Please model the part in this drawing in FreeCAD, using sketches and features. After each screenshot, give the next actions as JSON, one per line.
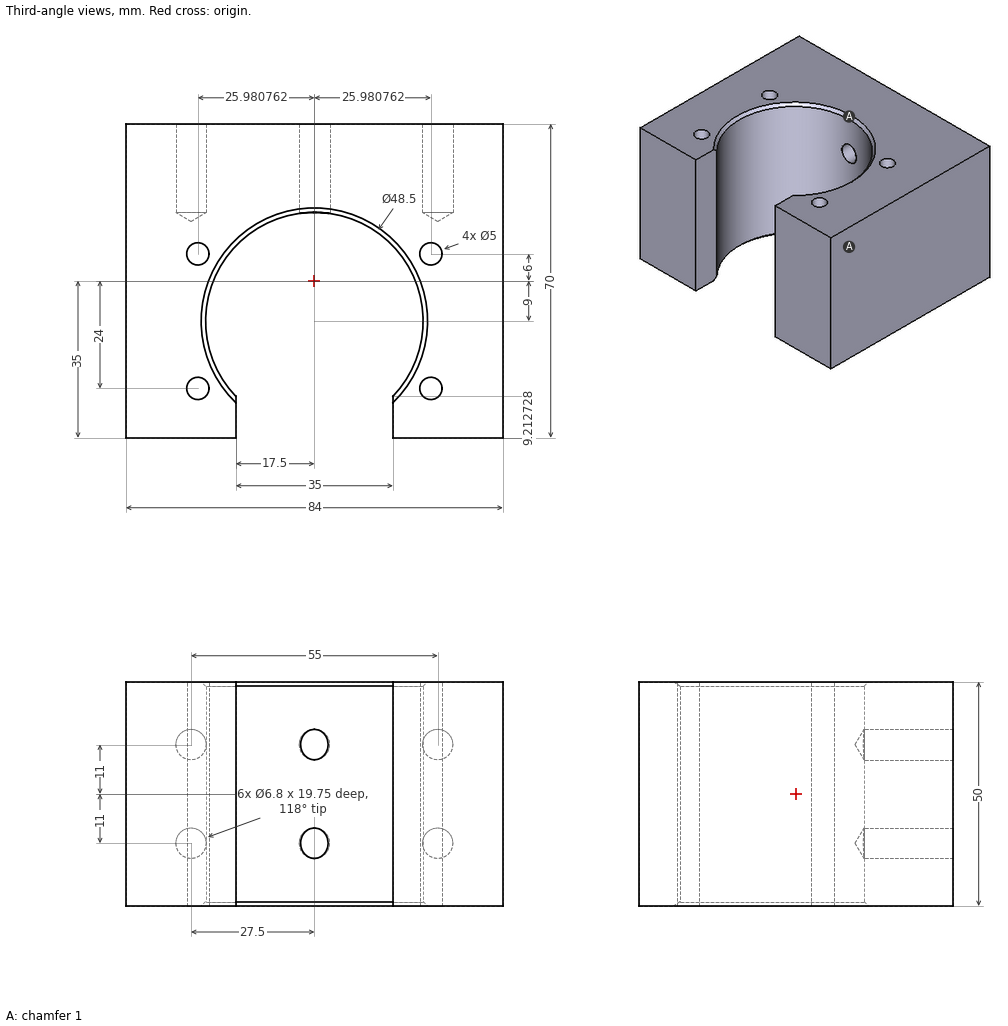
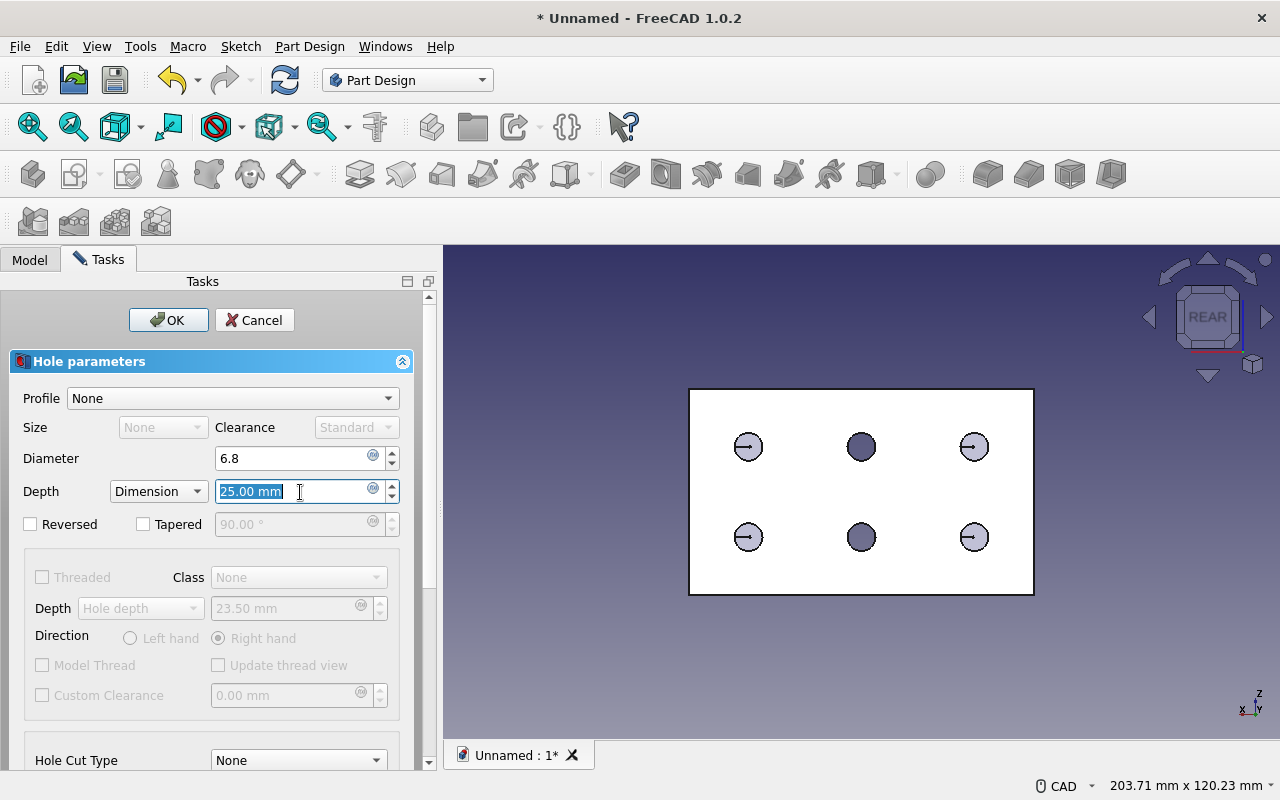
{"action": "type", "text": "19.75"}
{"action": "key", "text": "Tab"}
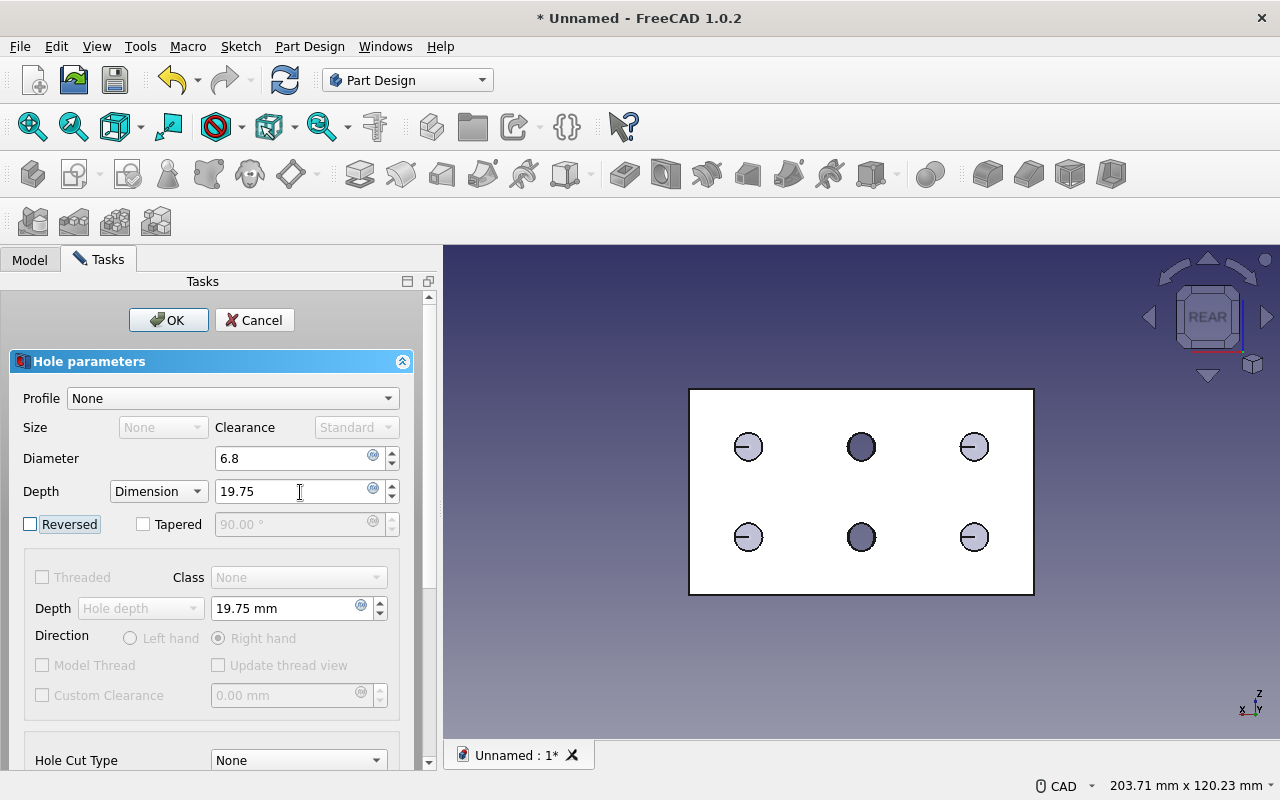
{"action": "left_click", "coordinate": [169, 320]}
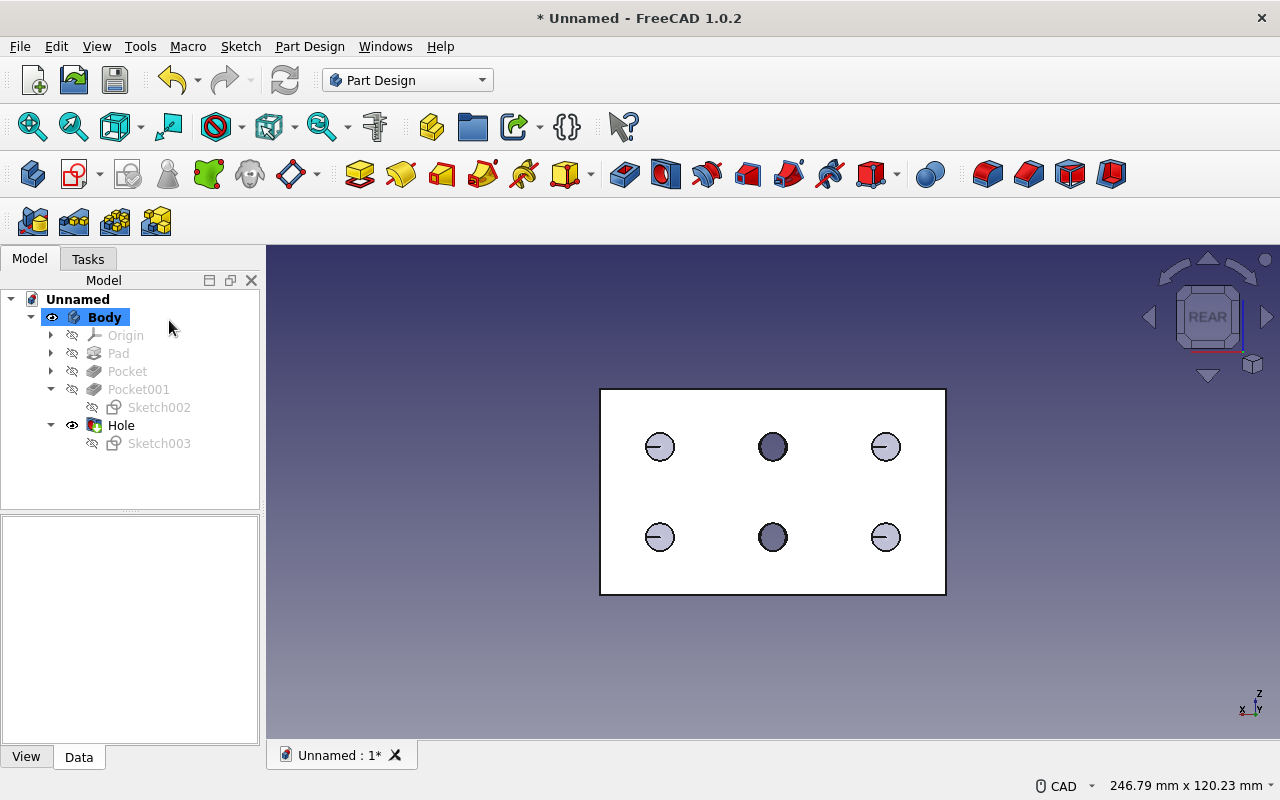
{"action": "key", "text": "v f"}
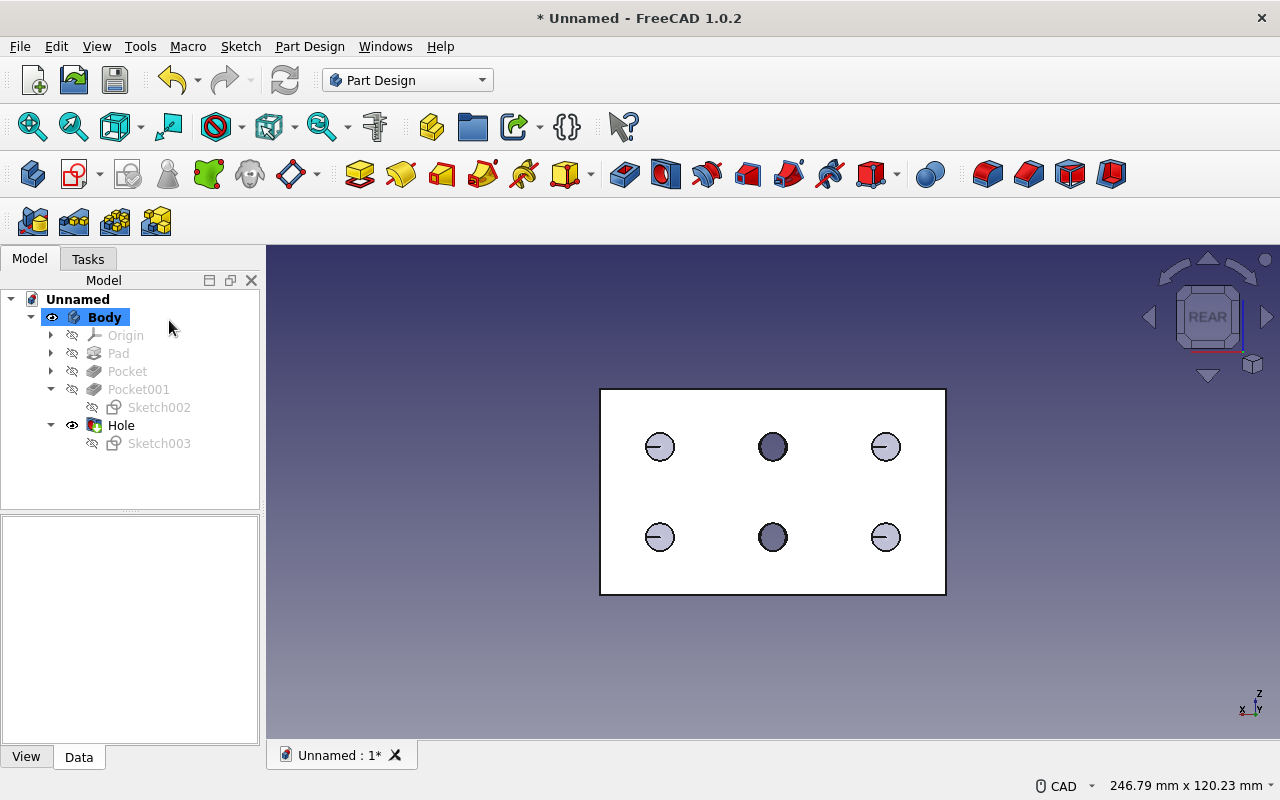
{"action": "key", "text": "0"}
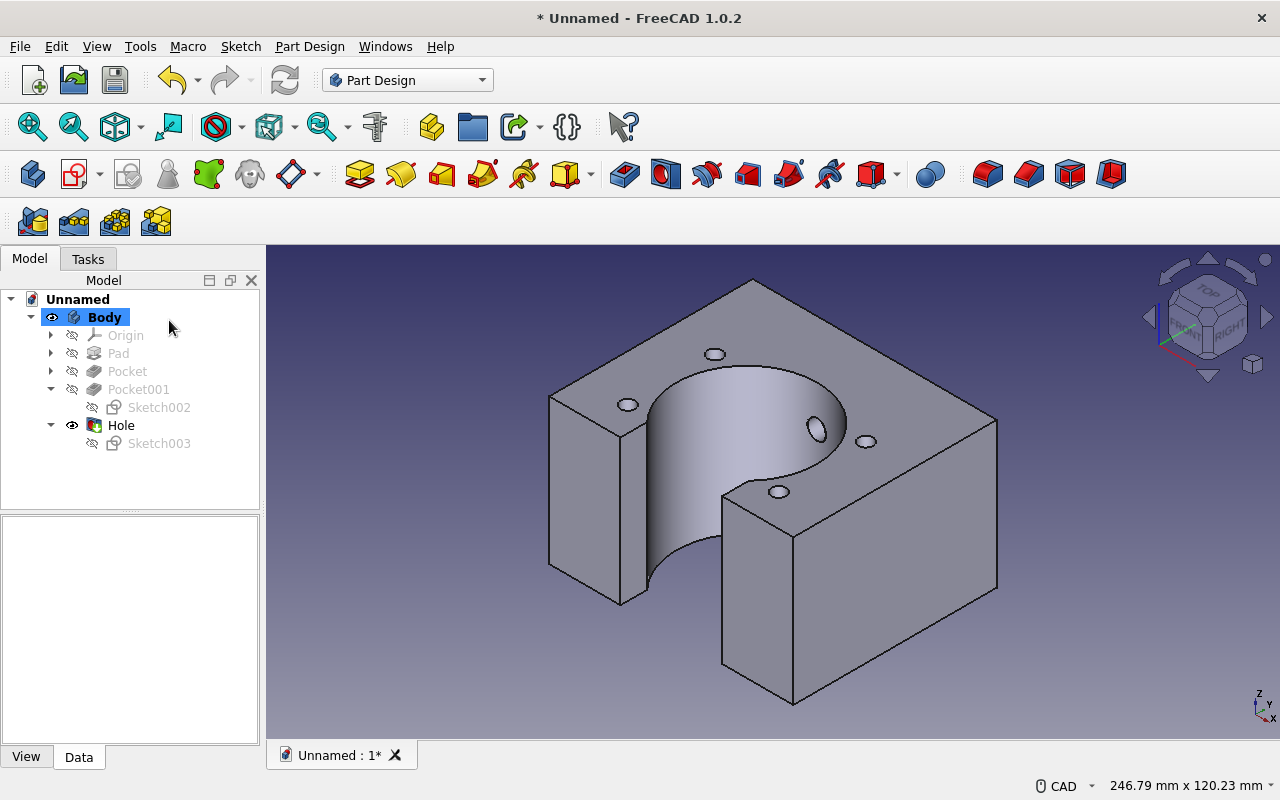
{"action": "left_click", "coordinate": [786, 369]}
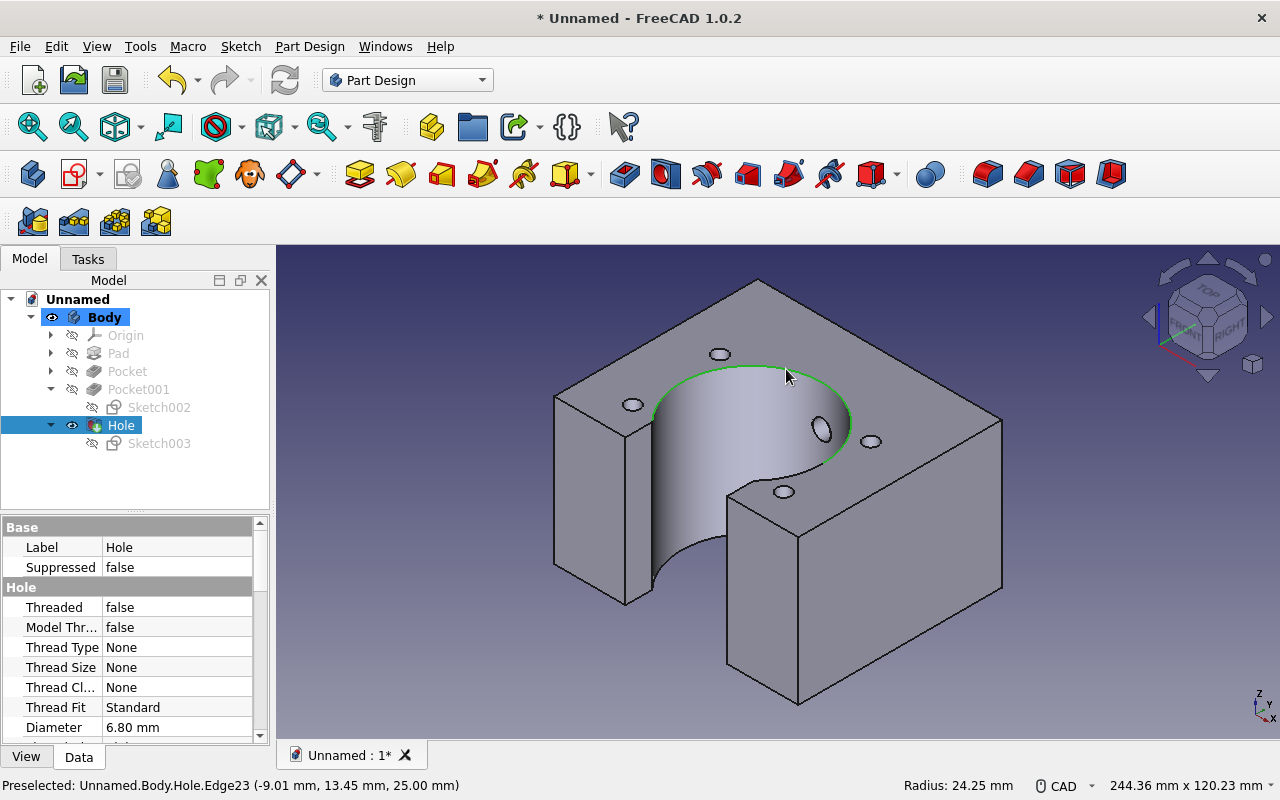
{"action": "key", "text": "2"}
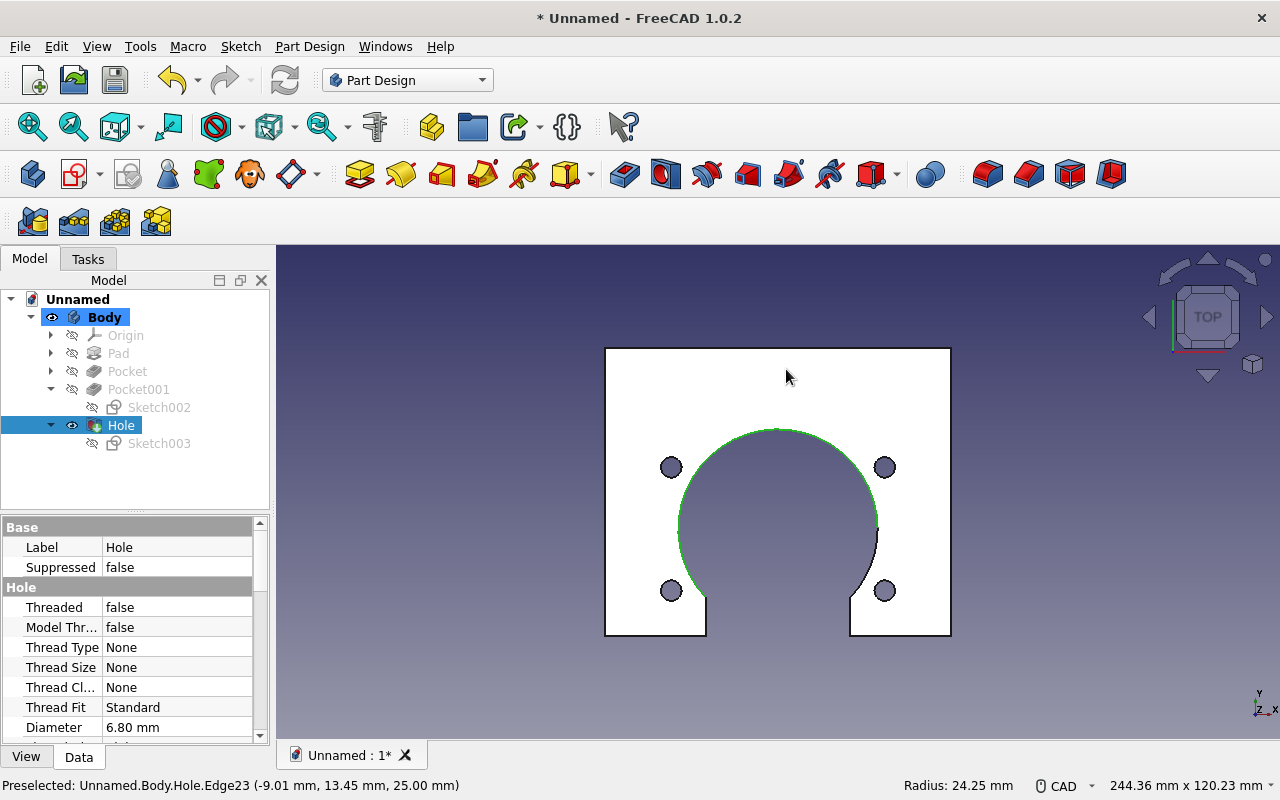
{"action": "key", "text": "1"}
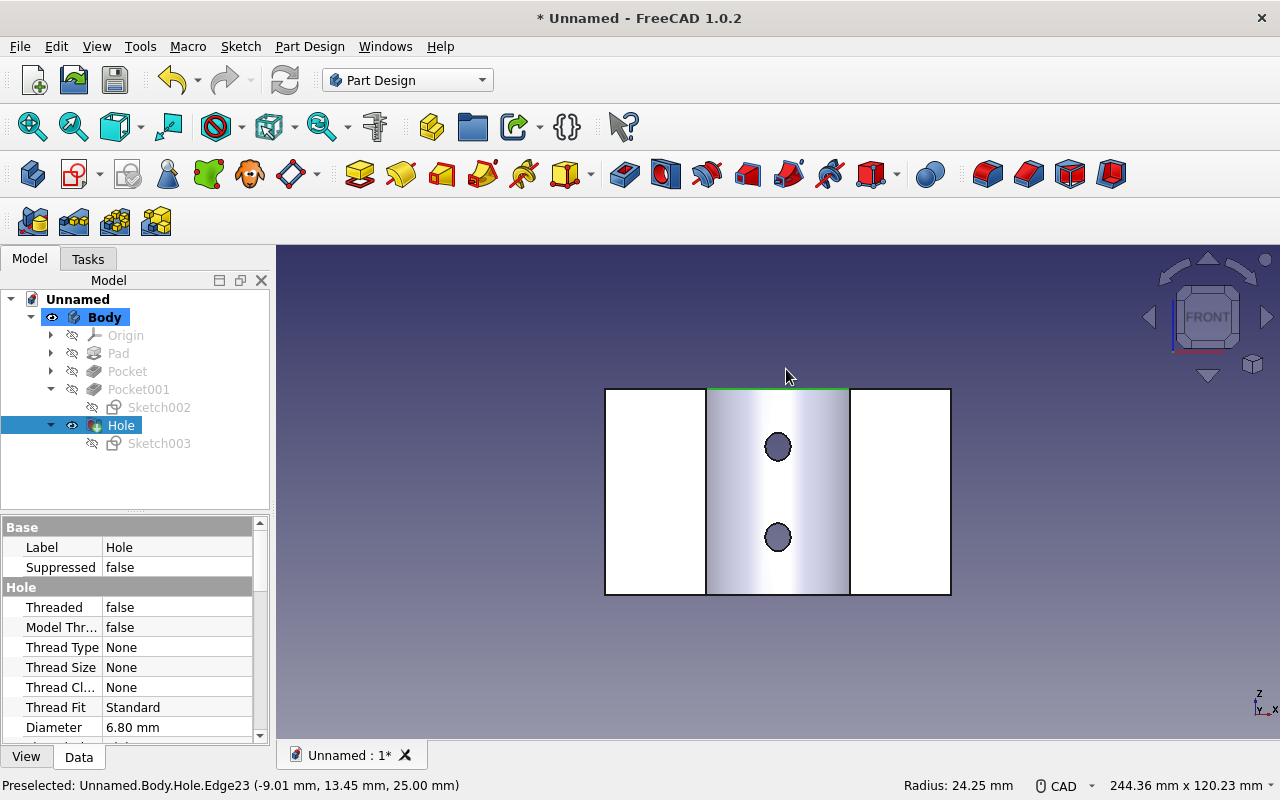
{"action": "left_click", "coordinate": [33, 128]}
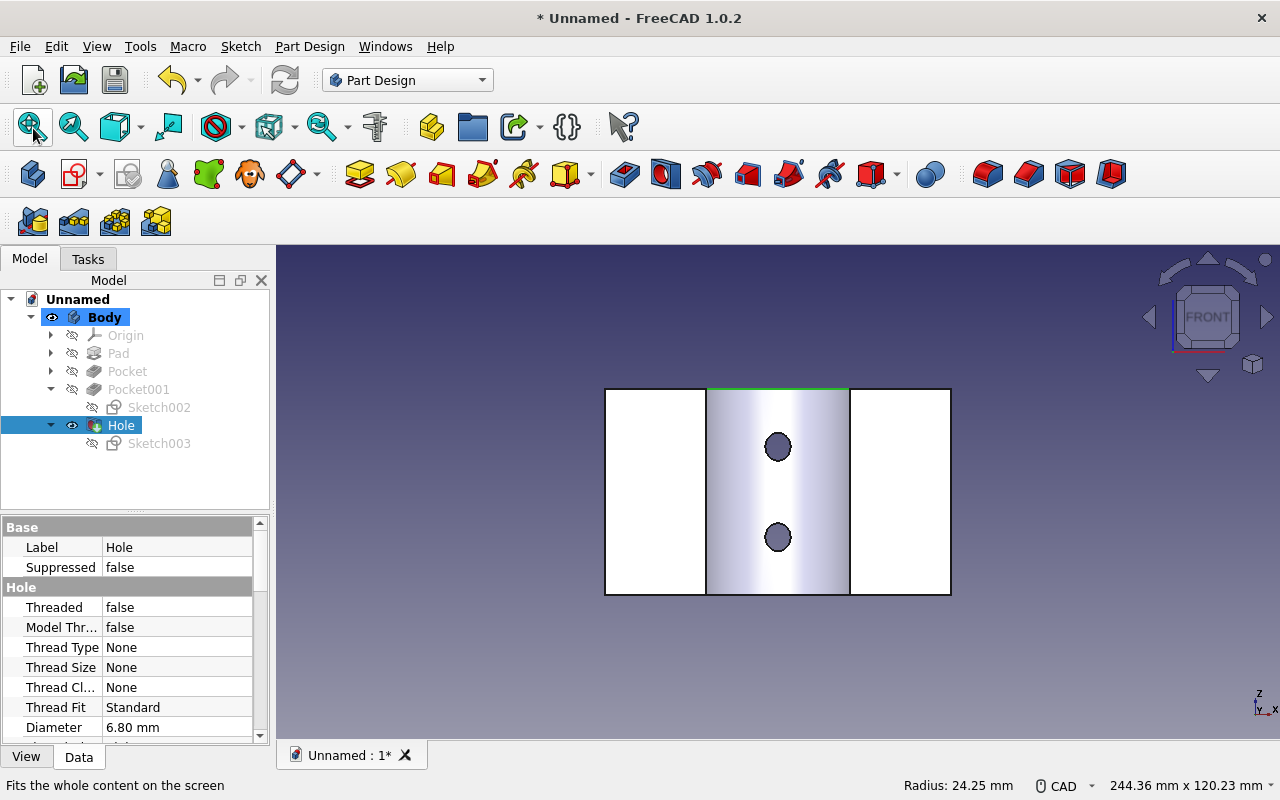
{"action": "left_click", "coordinate": [741, 594], "text": "ctrl"}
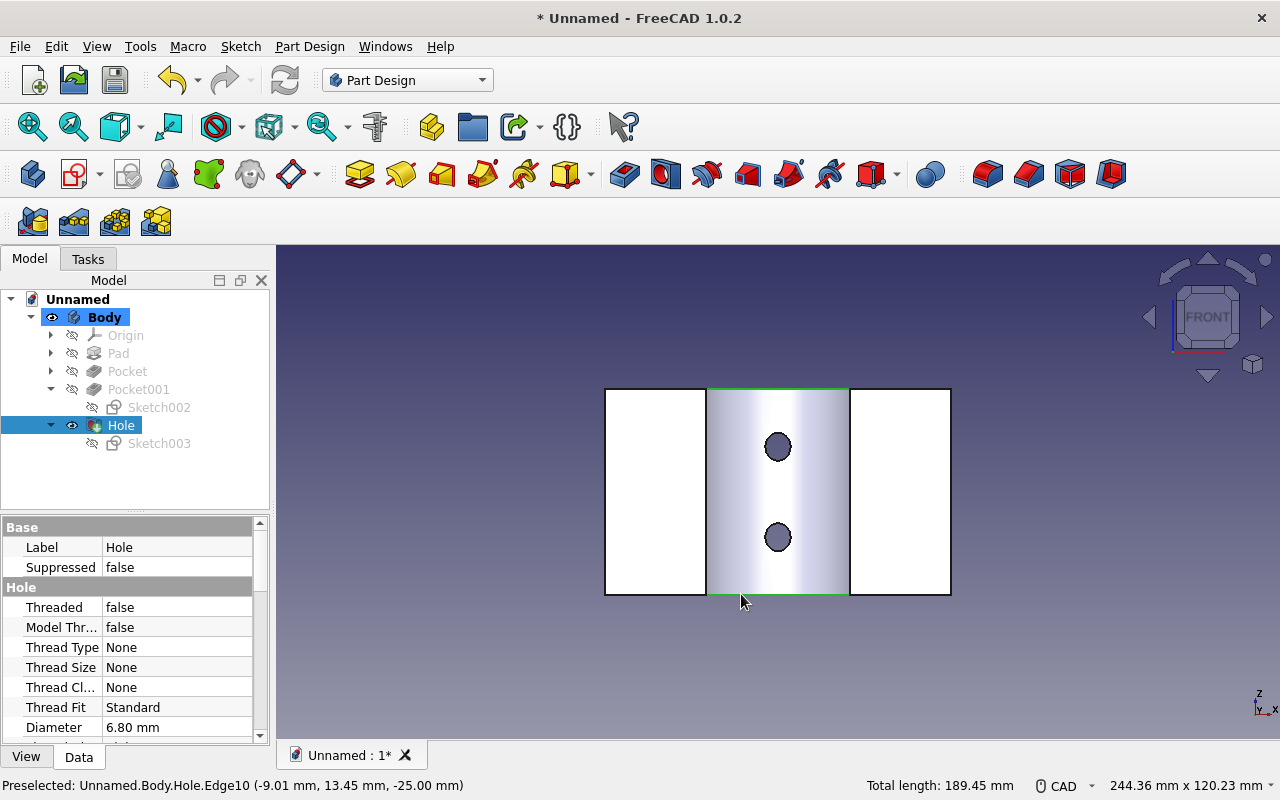
{"action": "left_click", "coordinate": [1029, 174]}